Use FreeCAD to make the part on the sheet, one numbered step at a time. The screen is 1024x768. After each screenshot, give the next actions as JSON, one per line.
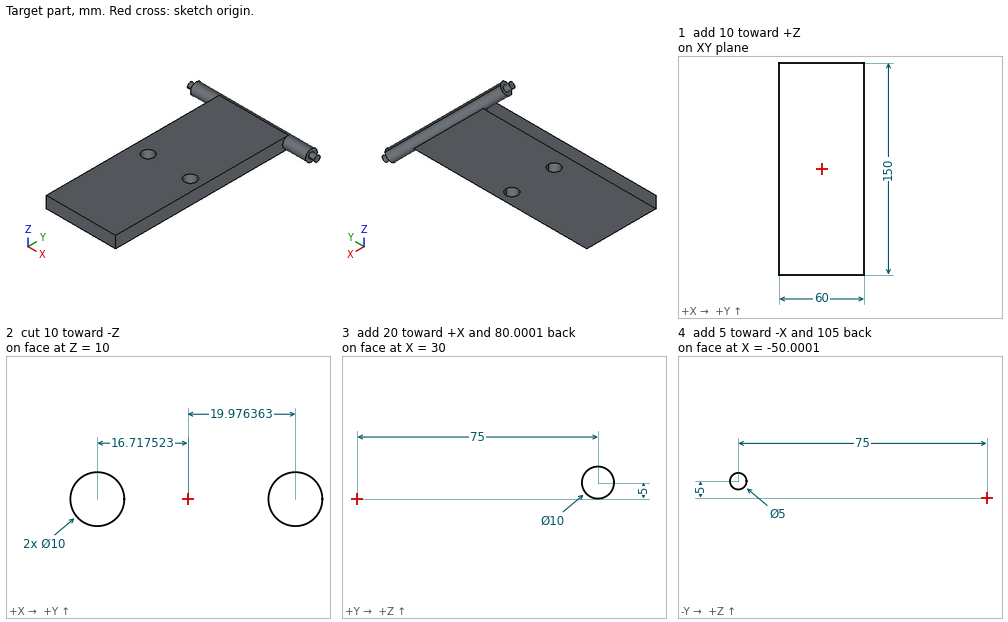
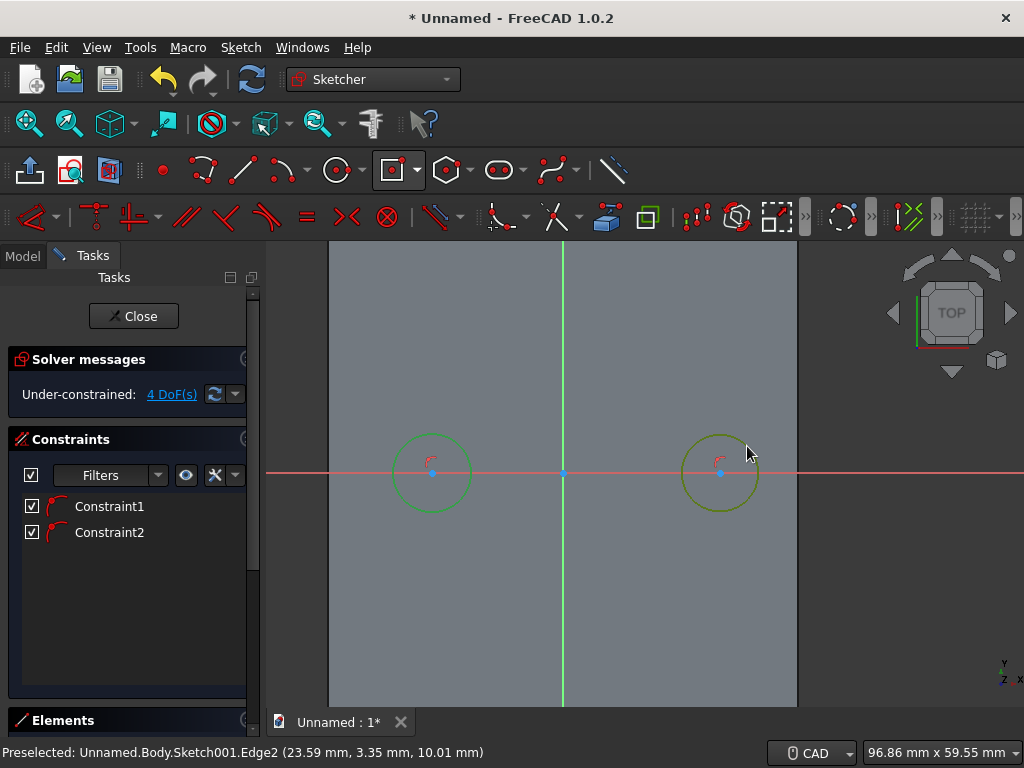
{"action": "left_click", "coordinate": [308, 218]}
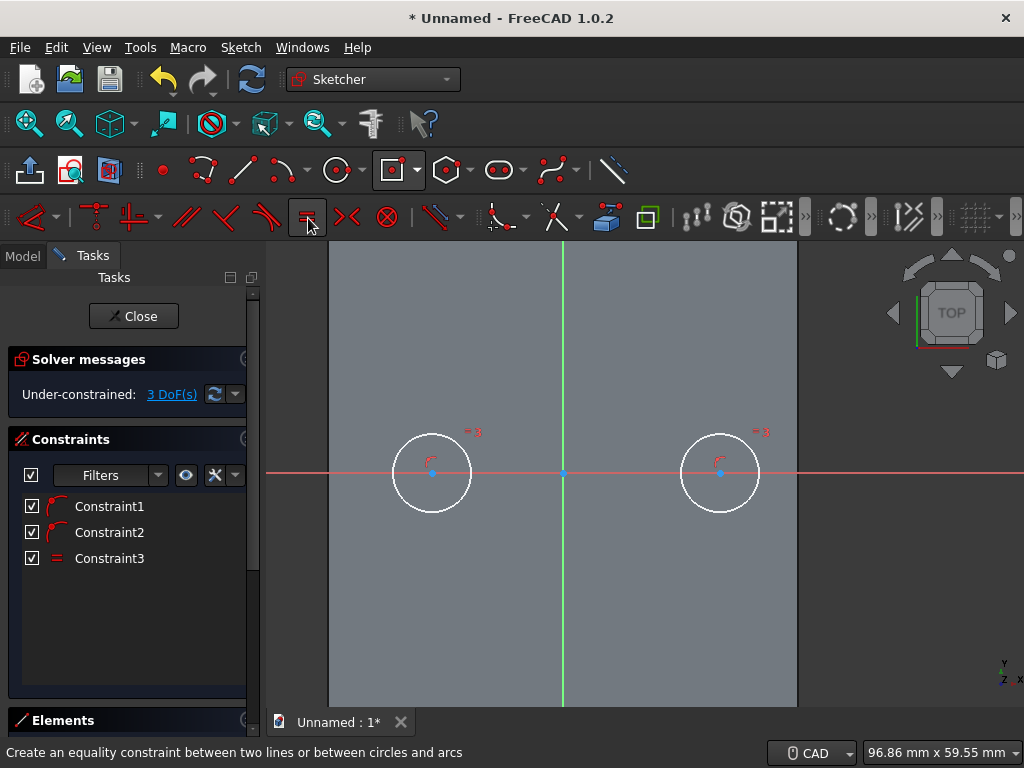
{"action": "left_click", "coordinate": [32, 218]}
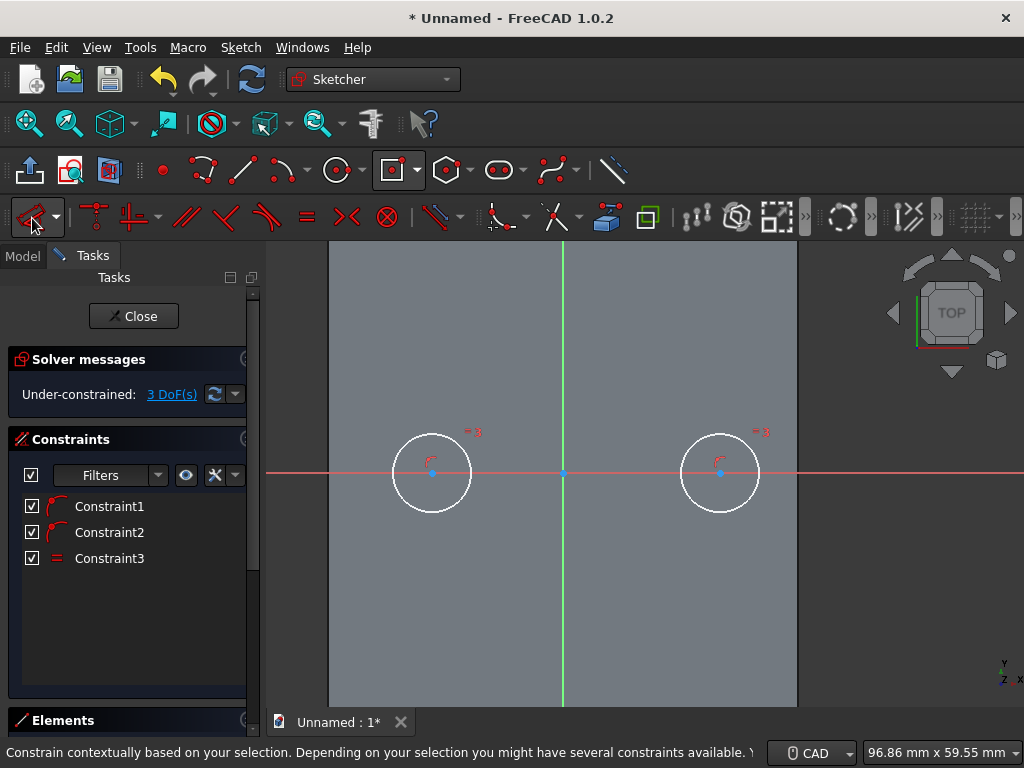
{"action": "left_click", "coordinate": [459, 445]}
{"action": "left_click", "coordinate": [481, 422]}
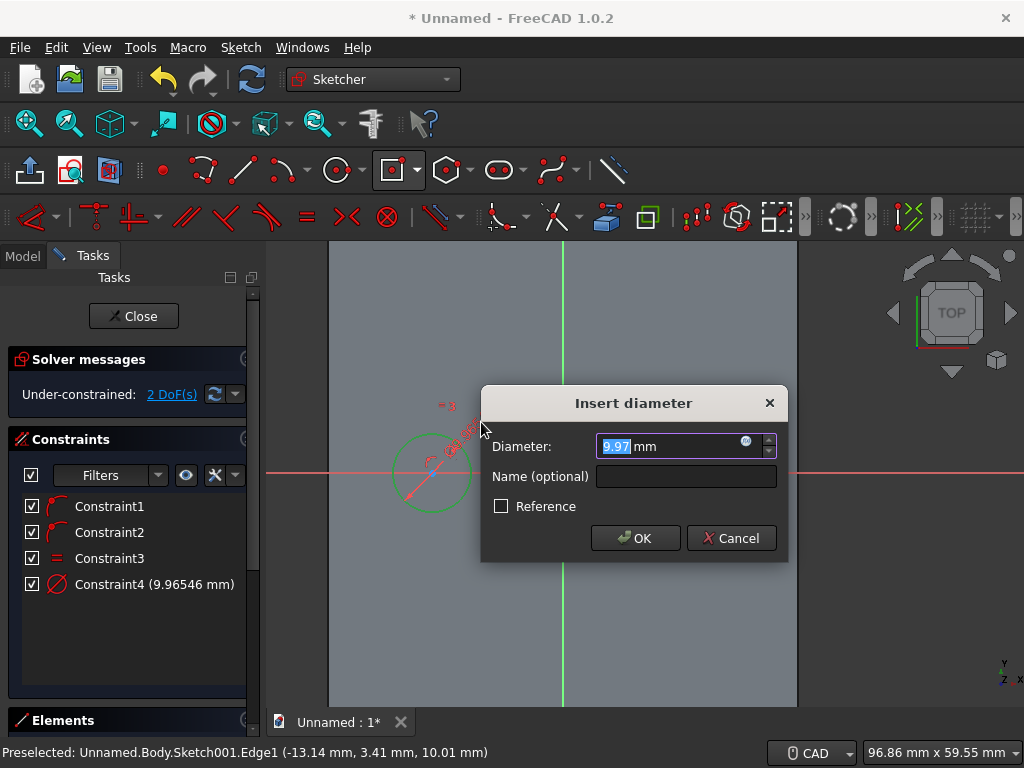
{"action": "type", "text": "10"}
{"action": "key", "text": "Return"}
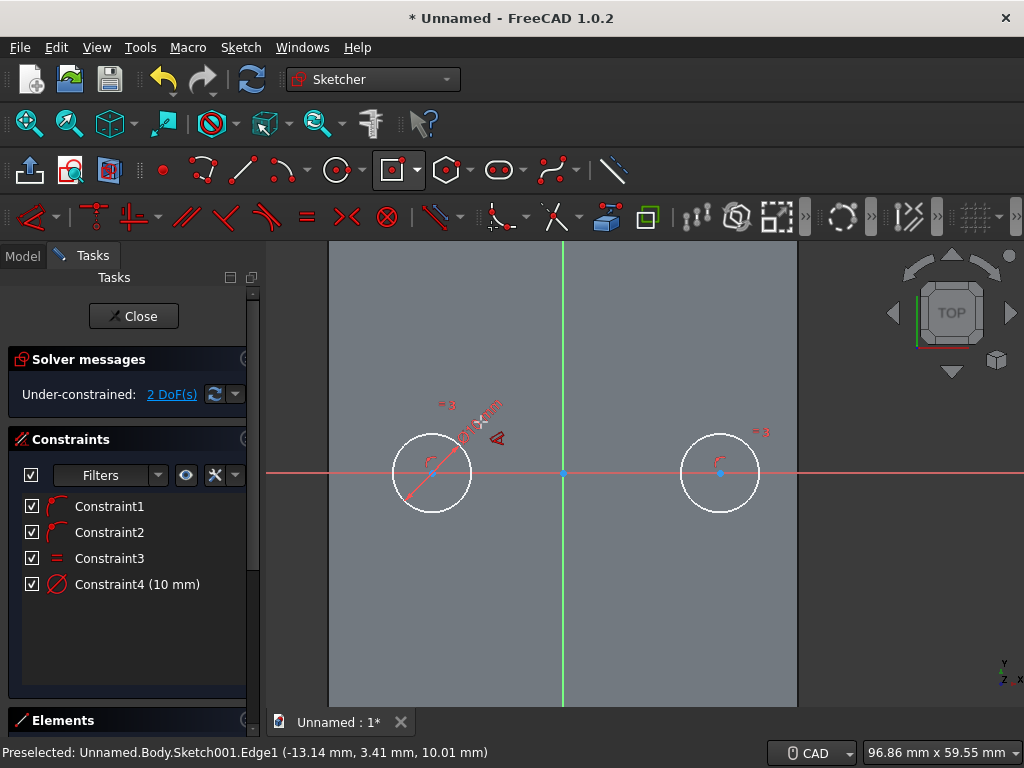
{"action": "left_click", "coordinate": [432, 473]}
{"action": "left_click", "coordinate": [498, 507]}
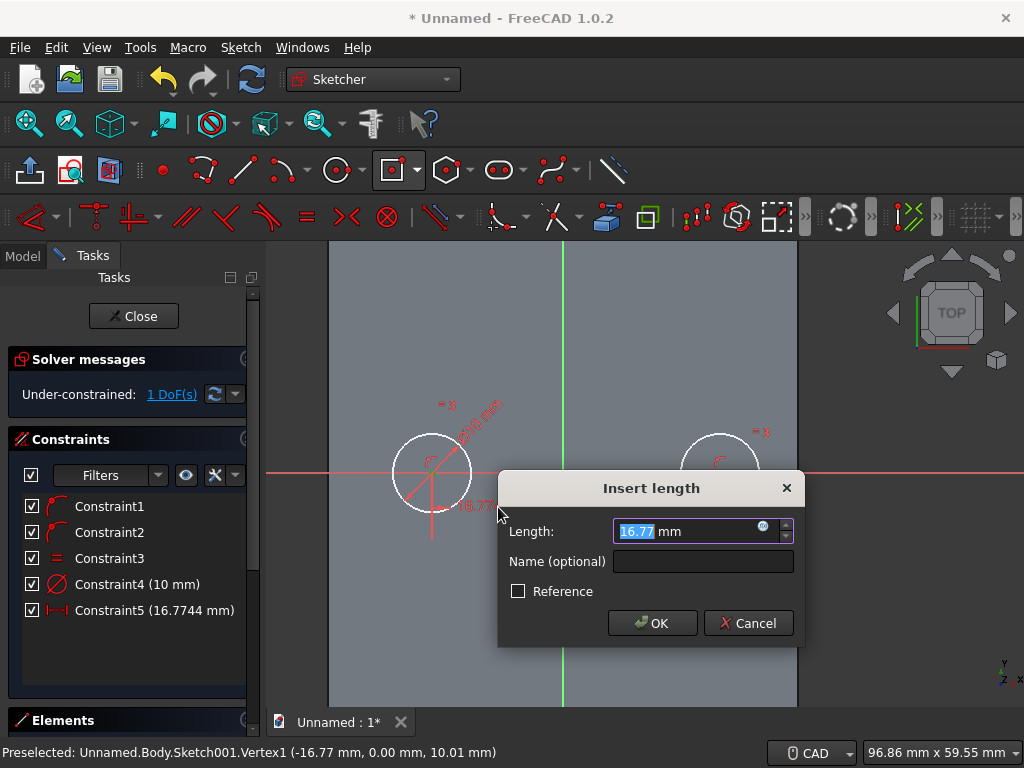
{"action": "type", "text": "16.717523"}
{"action": "key", "text": "Return"}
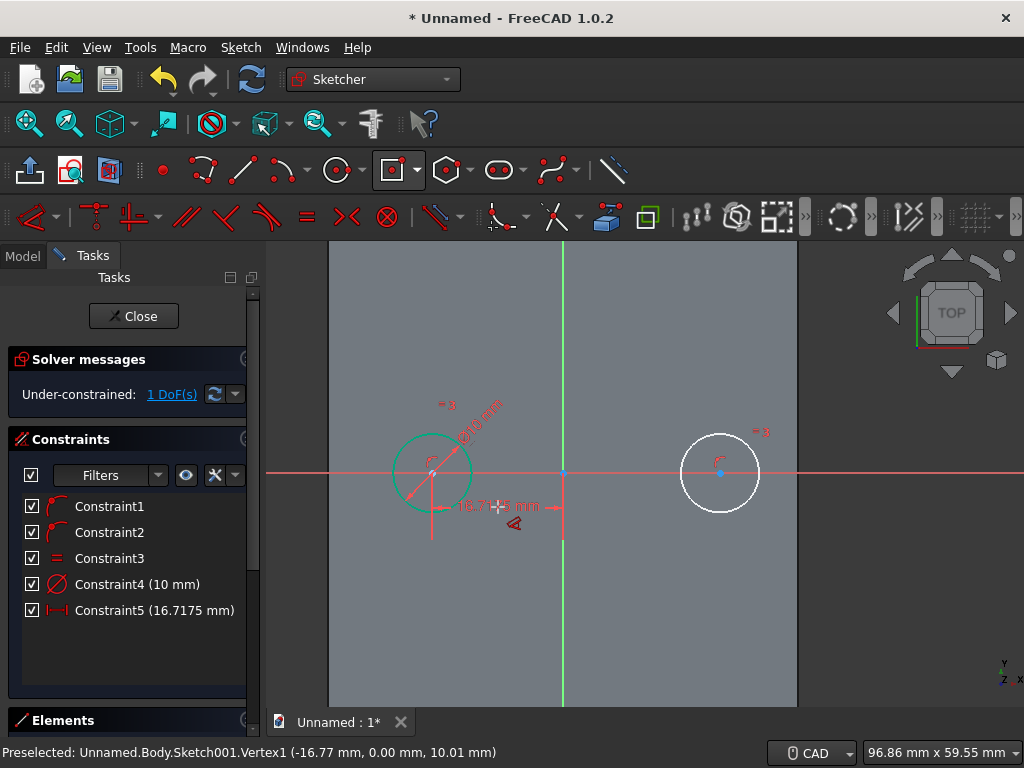
{"action": "left_click", "coordinate": [720, 473]}
{"action": "left_click", "coordinate": [642, 507]}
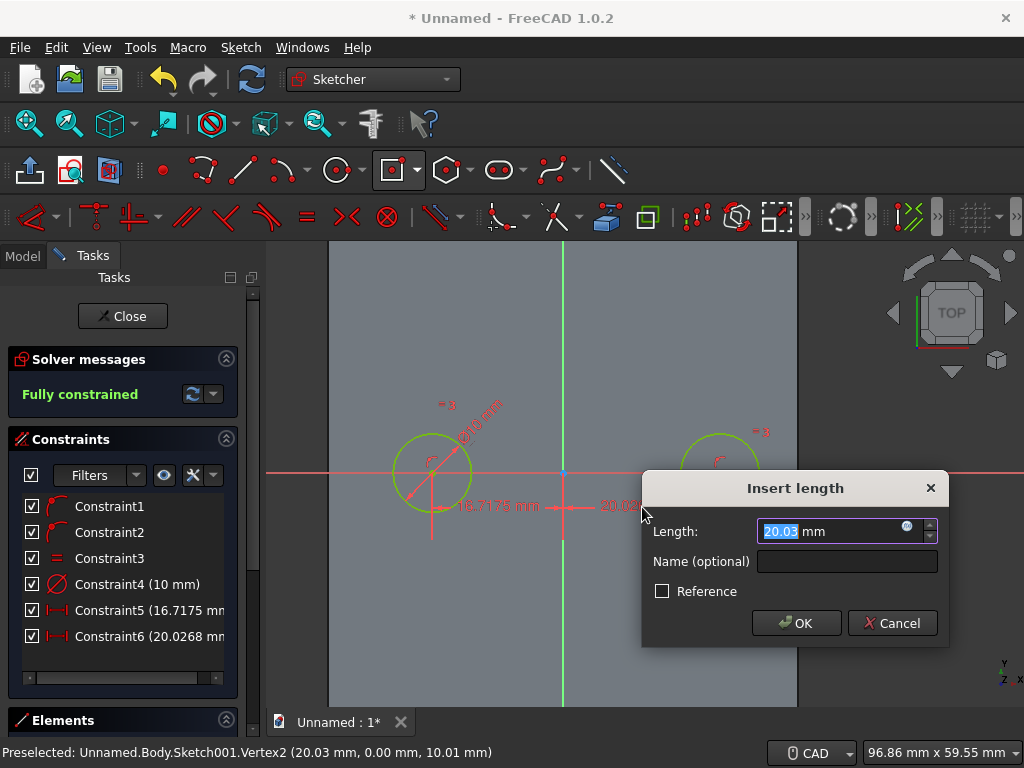
{"action": "type", "text": "19.976363"}
{"action": "key", "text": "Return"}
{"action": "key", "text": "Escape"}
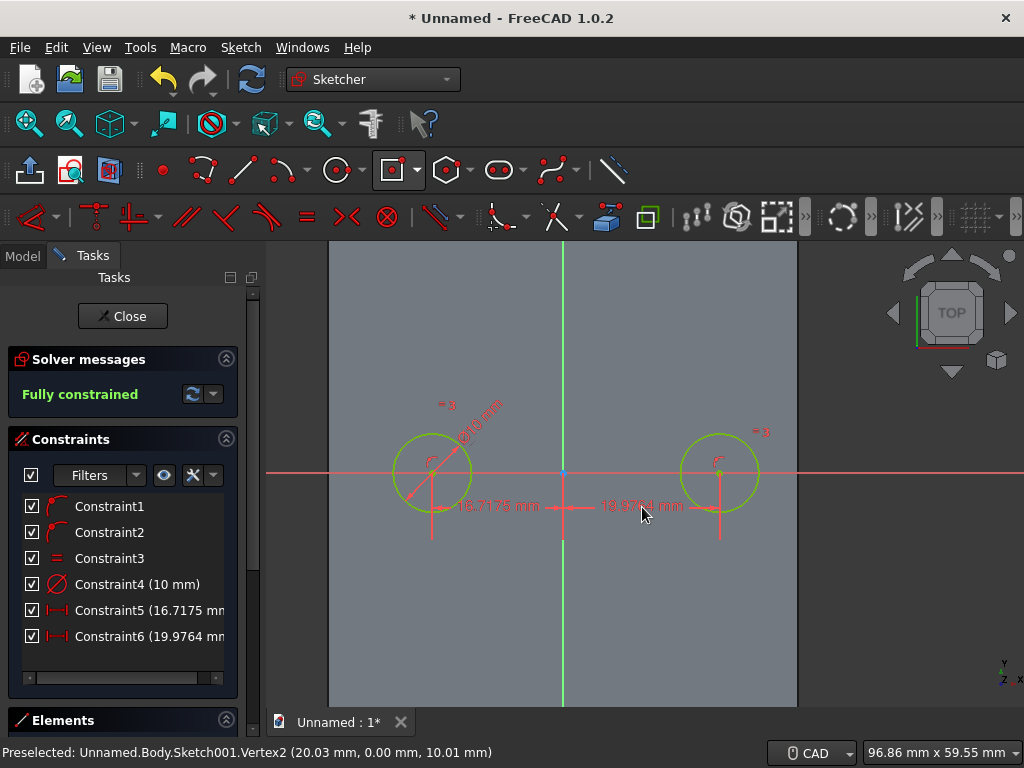
{"action": "left_click", "coordinate": [123, 316]}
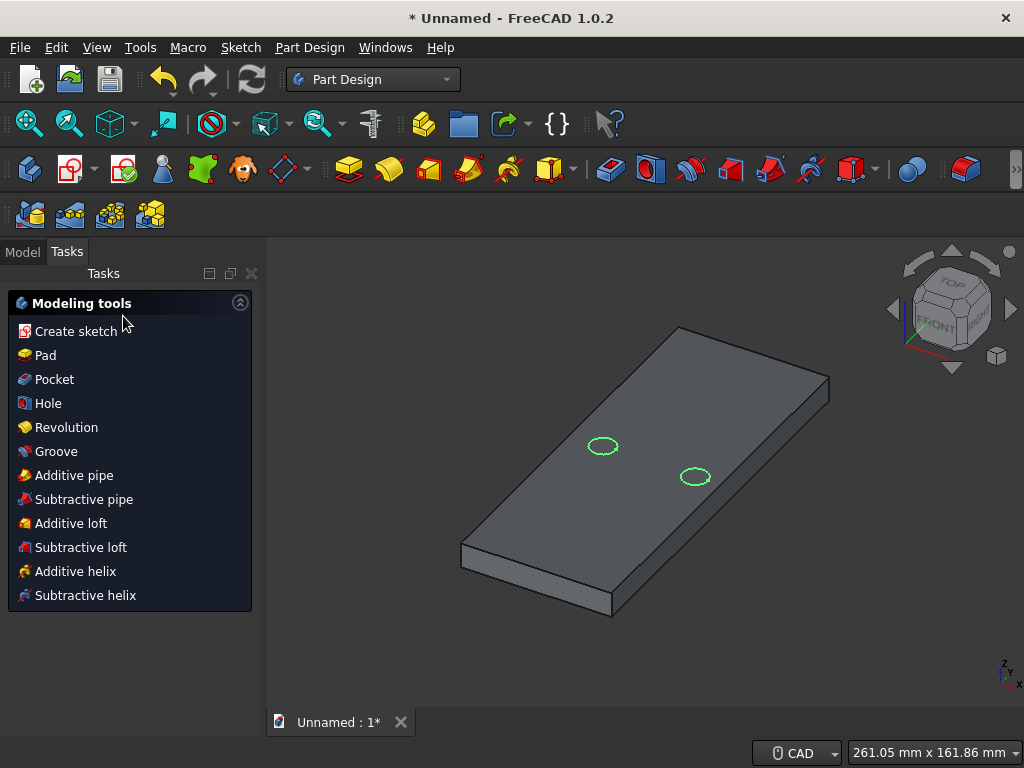
{"action": "left_click", "coordinate": [612, 170]}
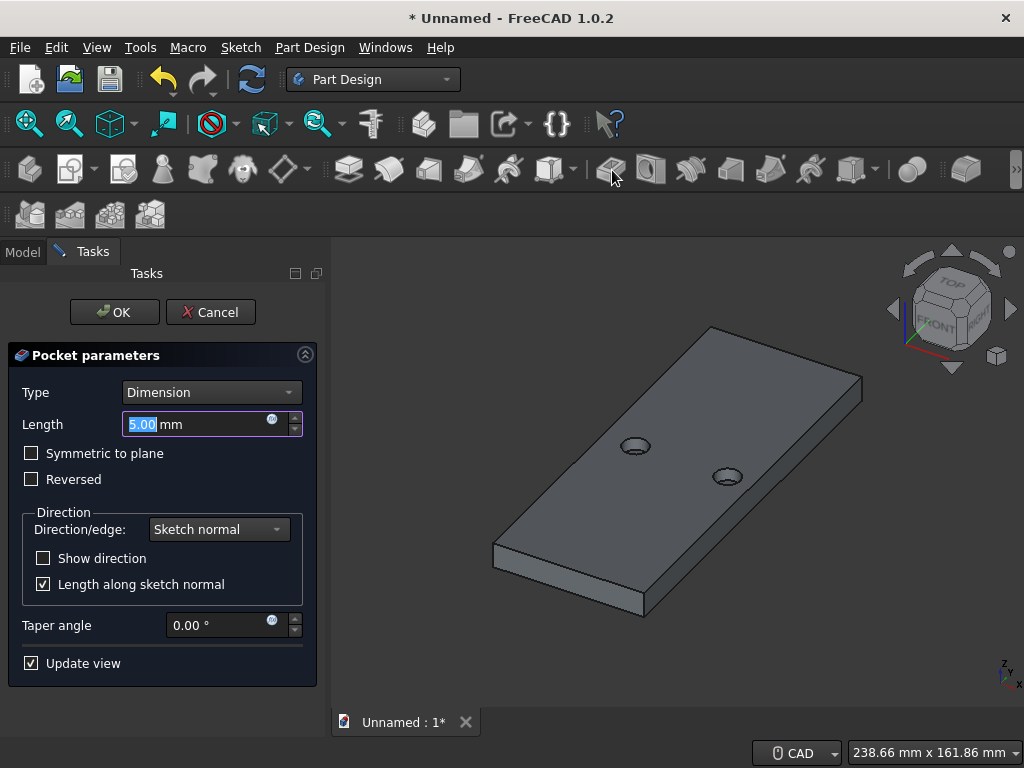
{"action": "type", "text": "10"}
{"action": "key", "text": "Tab"}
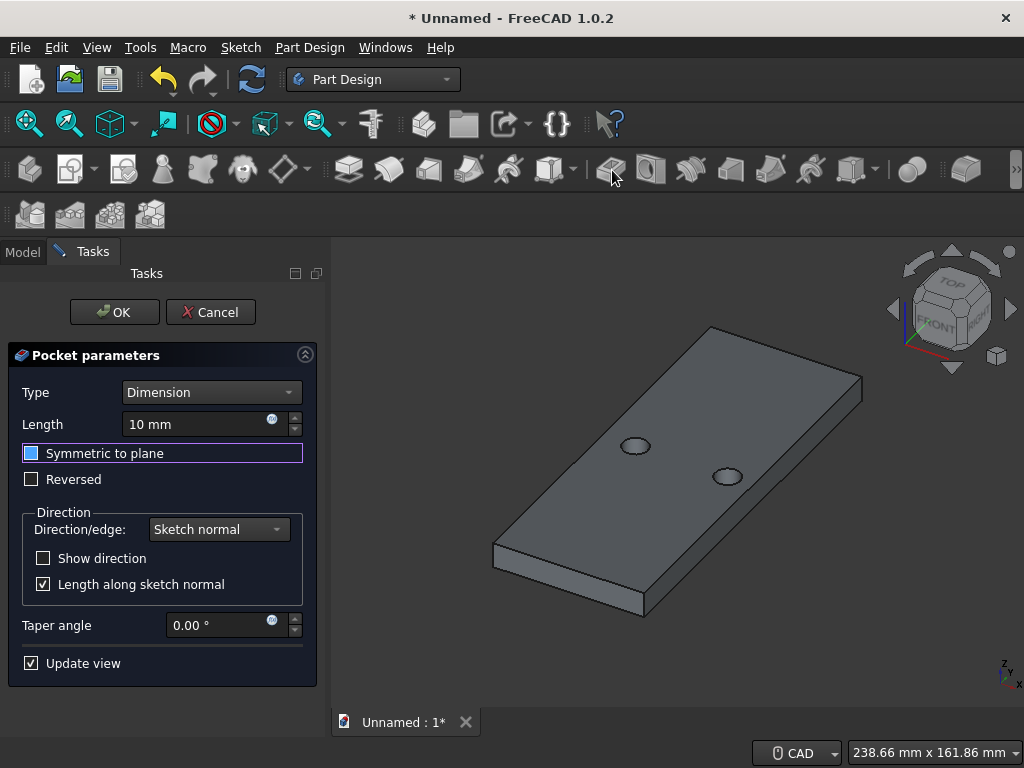
{"action": "left_click", "coordinate": [115, 312]}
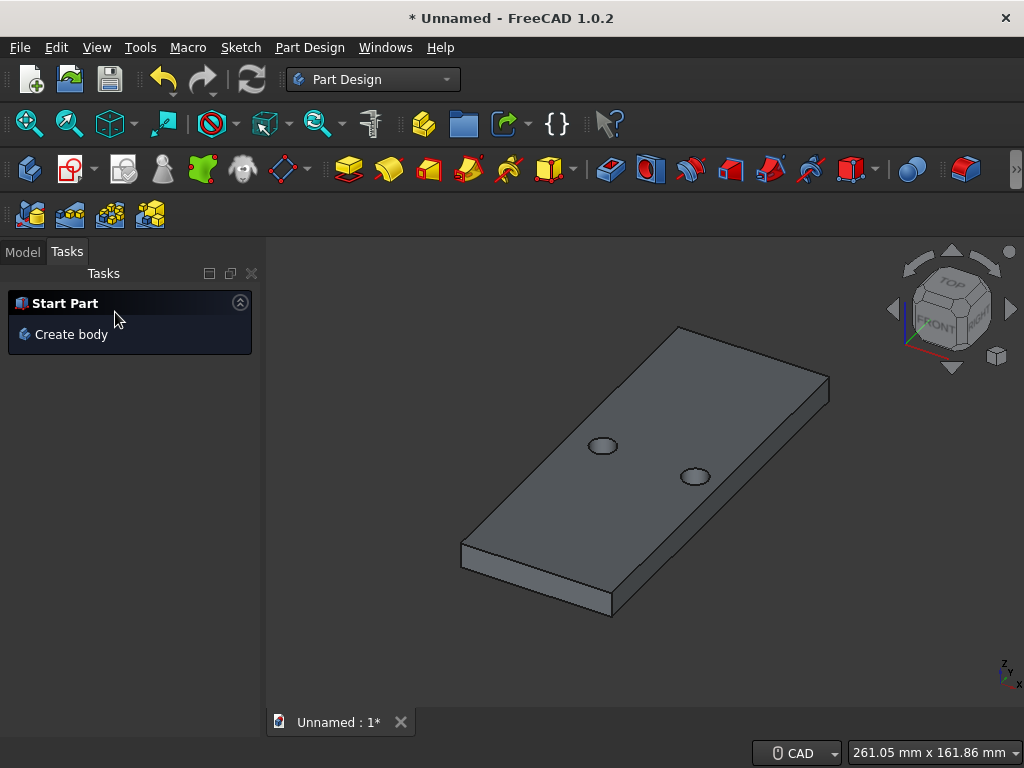
{"action": "key", "text": "0"}